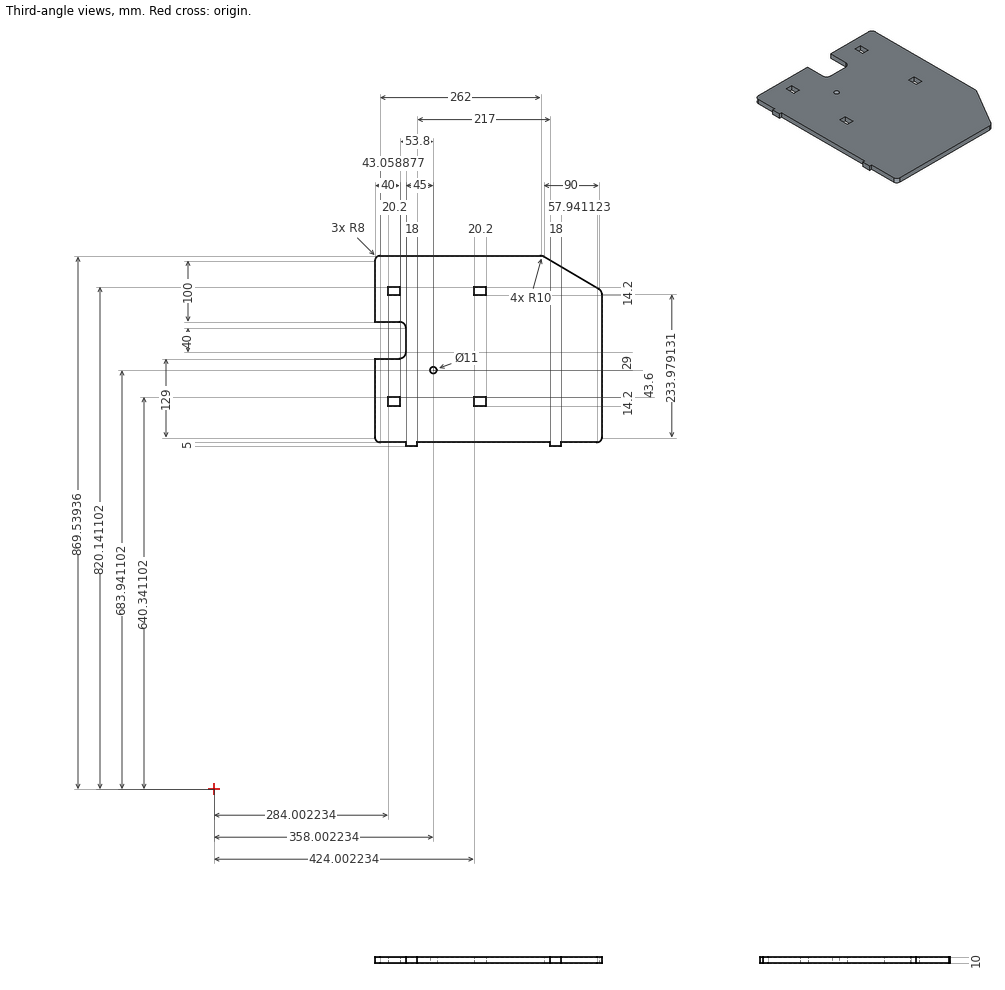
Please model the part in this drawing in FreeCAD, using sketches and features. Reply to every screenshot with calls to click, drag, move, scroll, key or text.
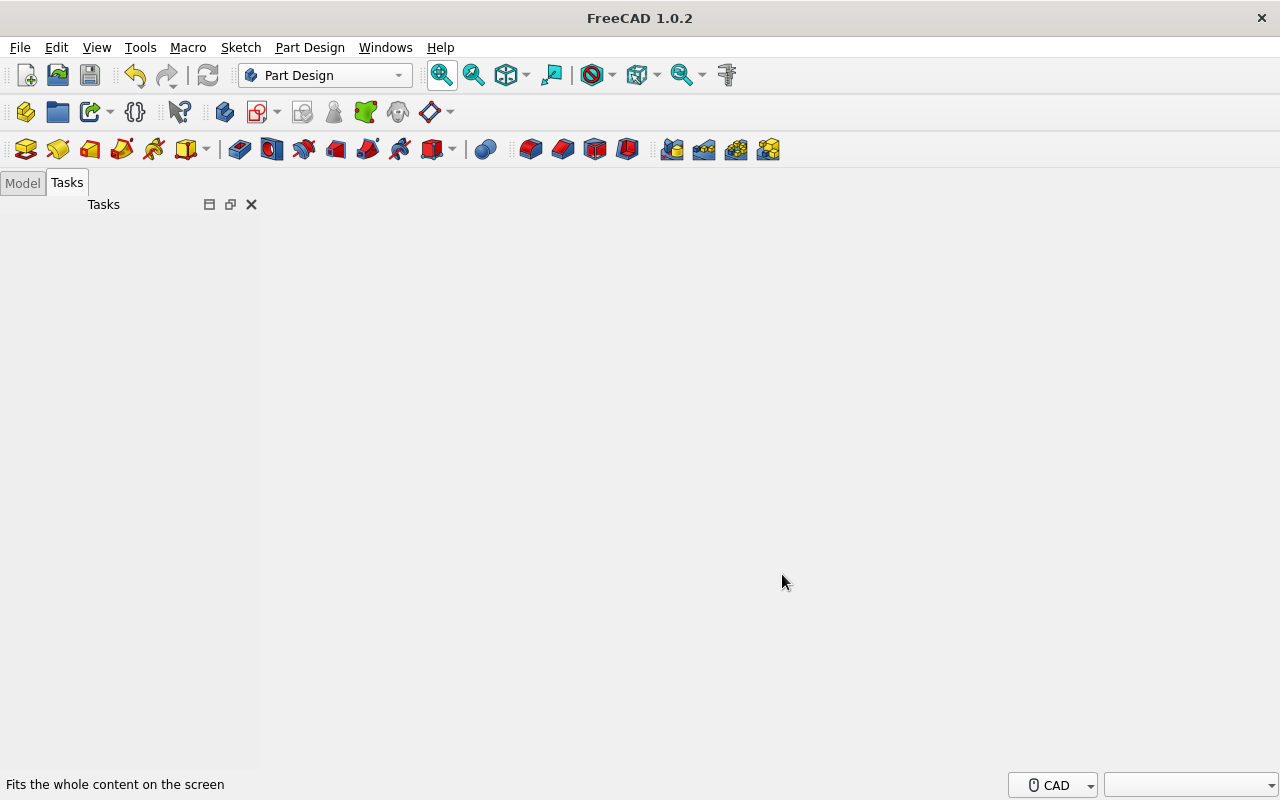
click(26, 76)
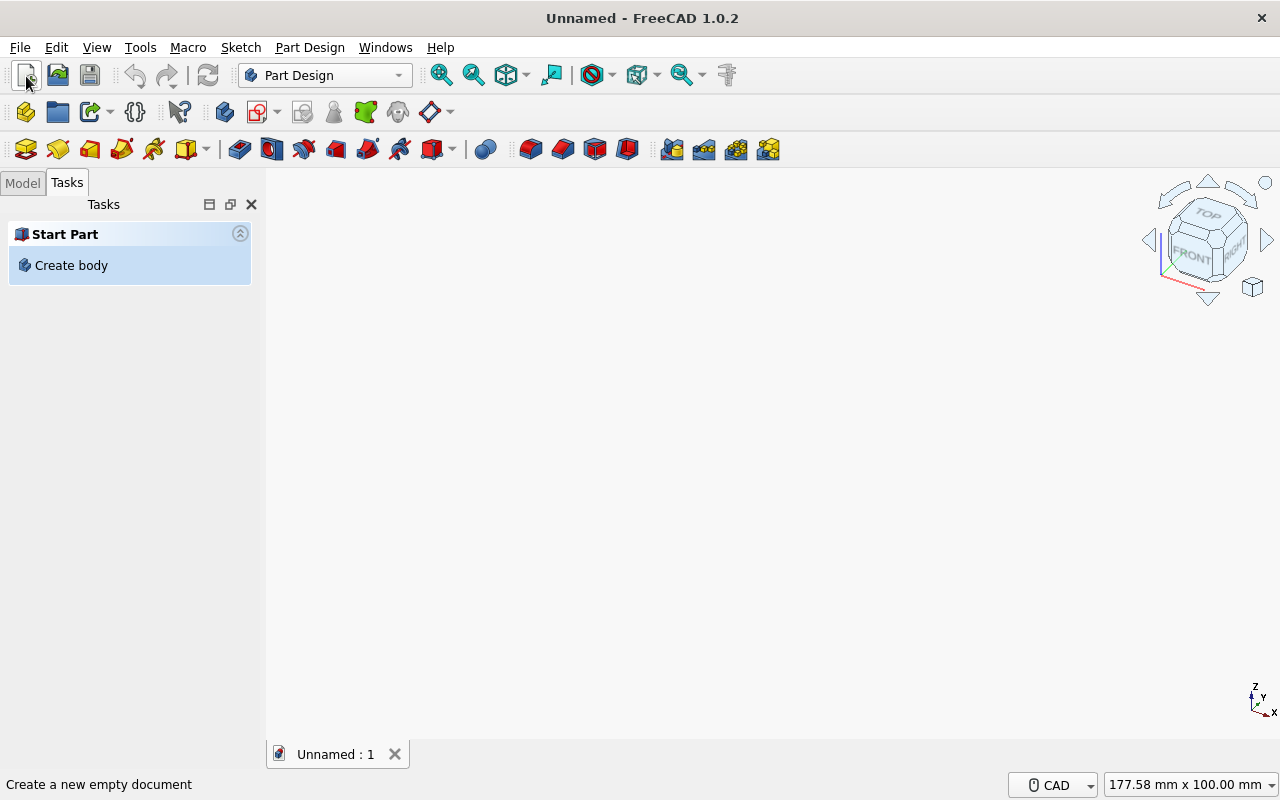
click(258, 112)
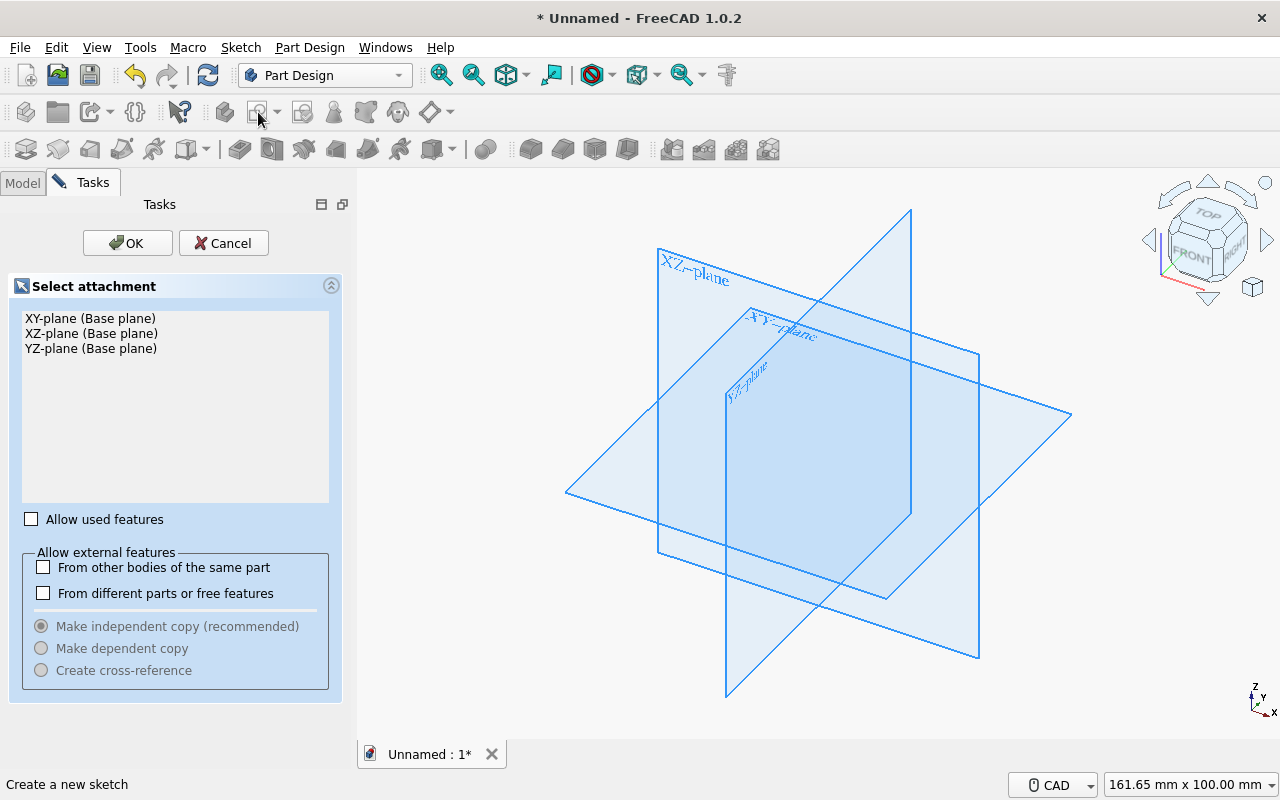
click(82, 318)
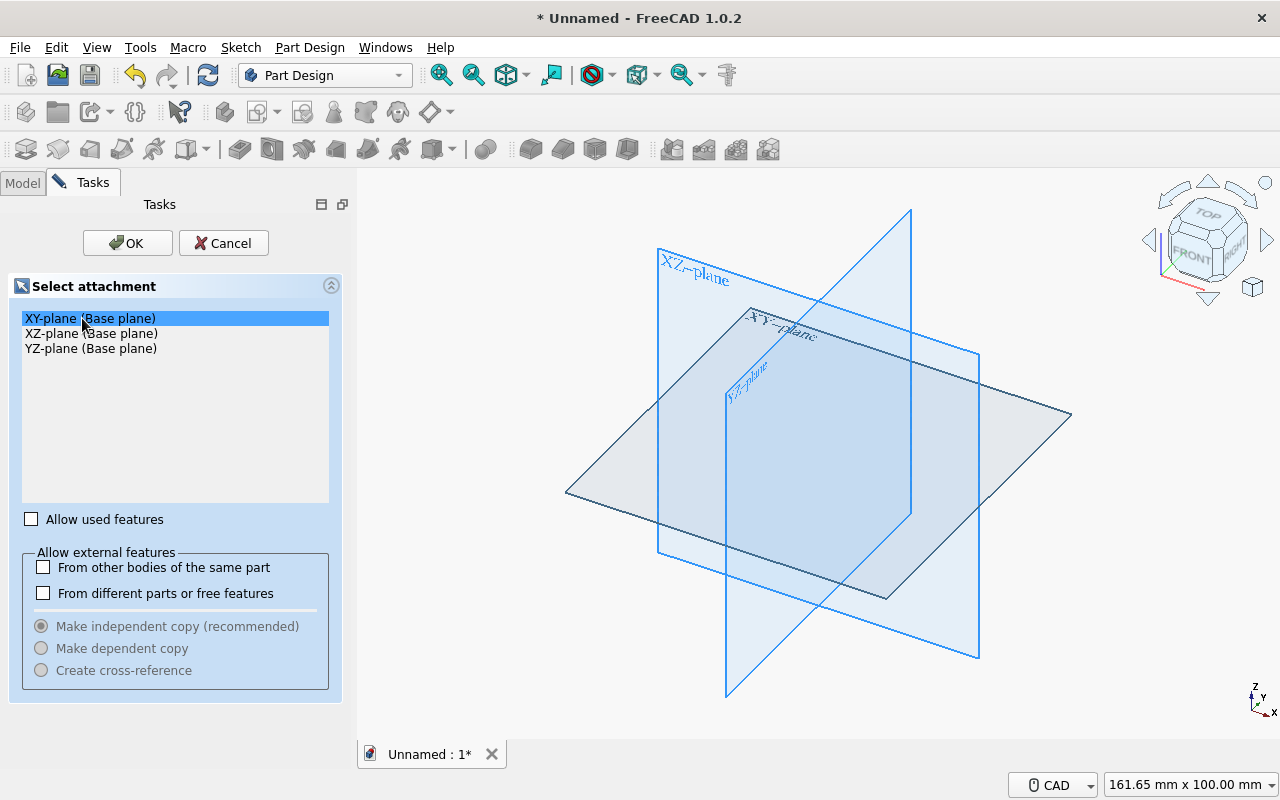
click(128, 243)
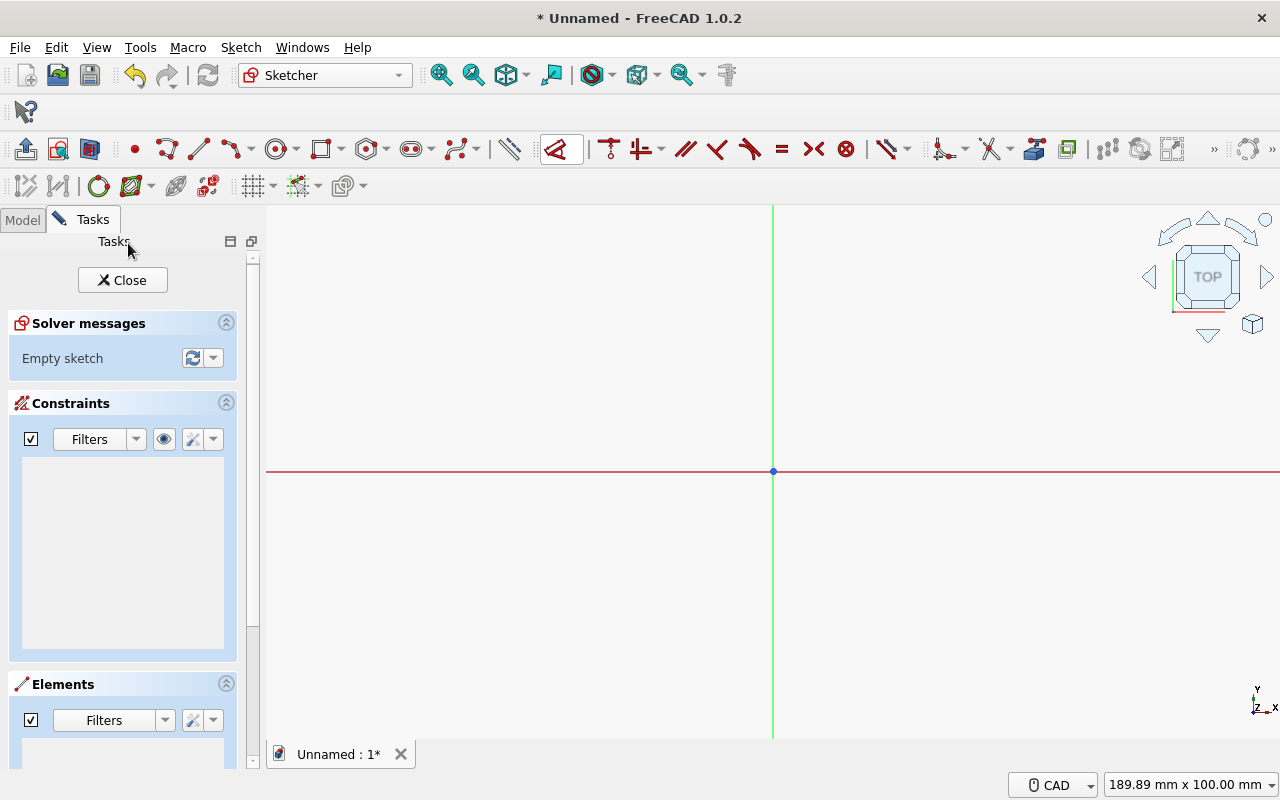
scroll(563, 659, down, 13)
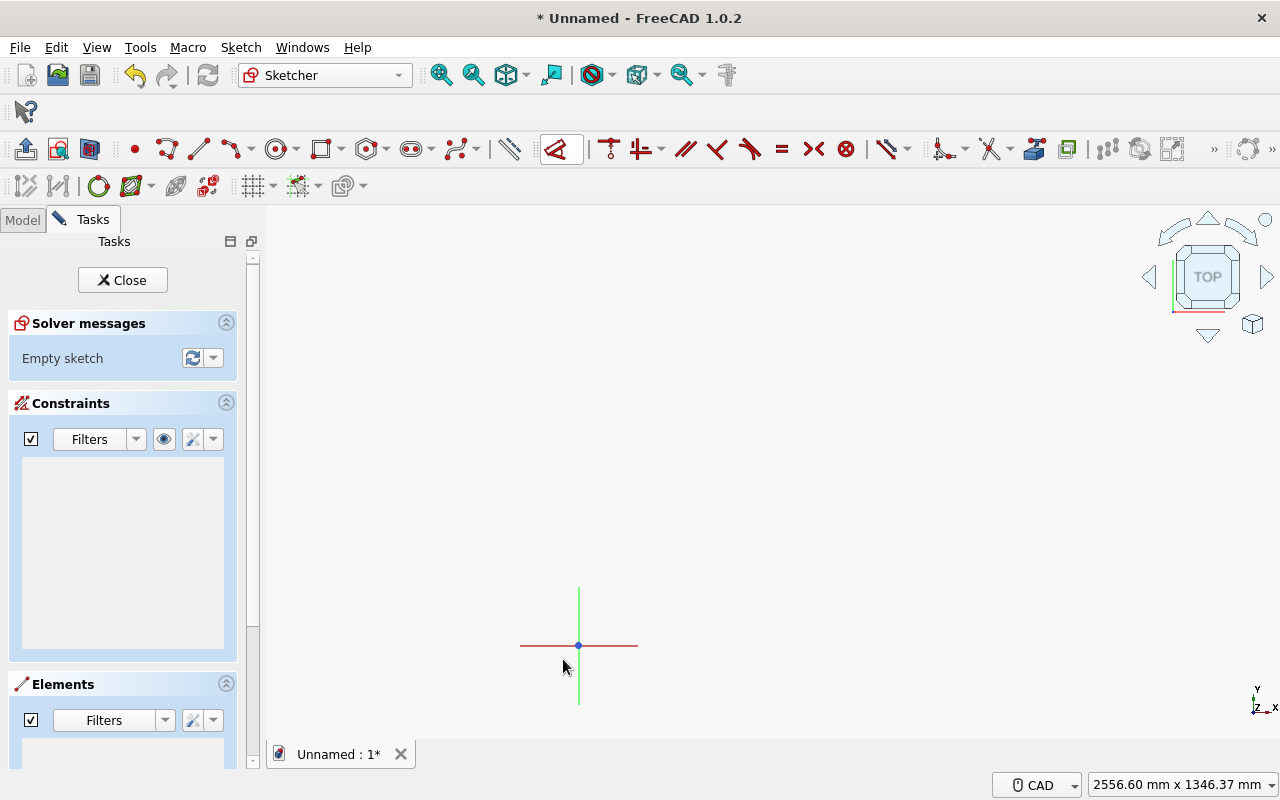
click(200, 150)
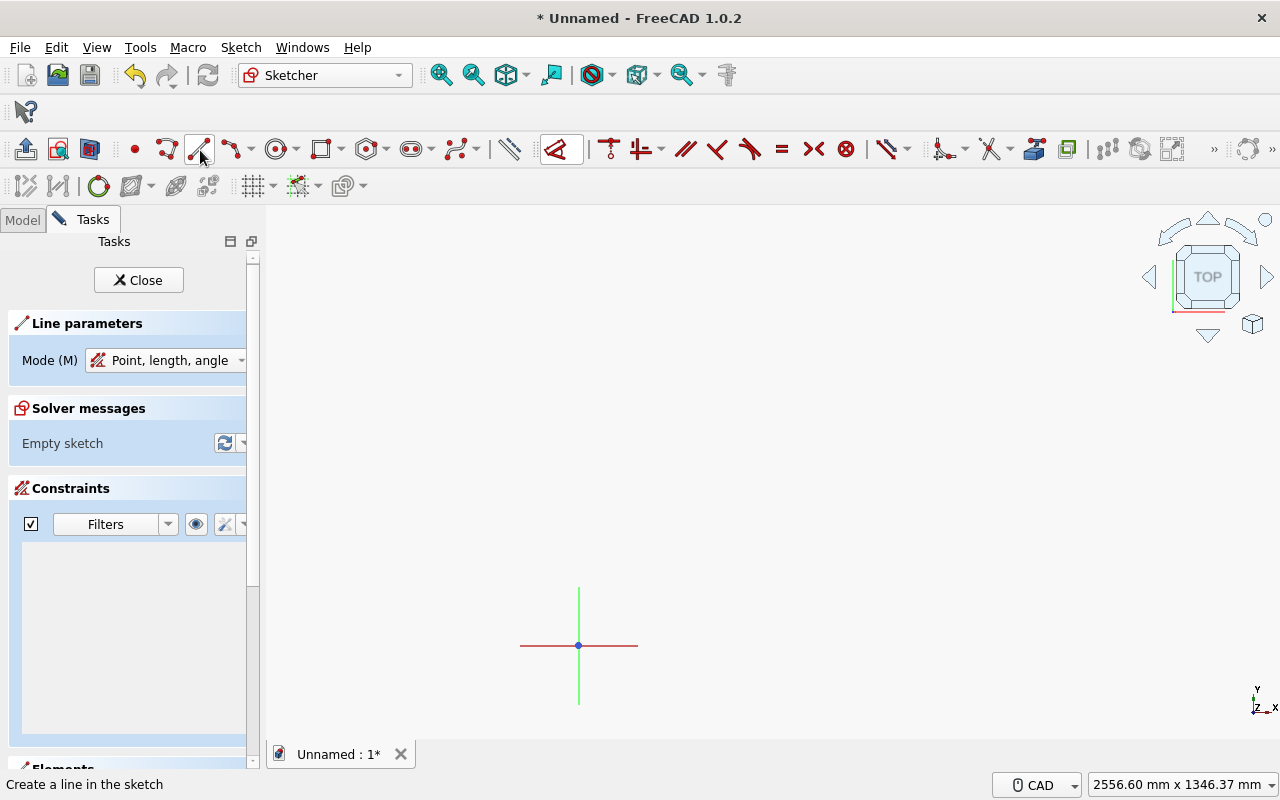
click(828, 322)
click(792, 301)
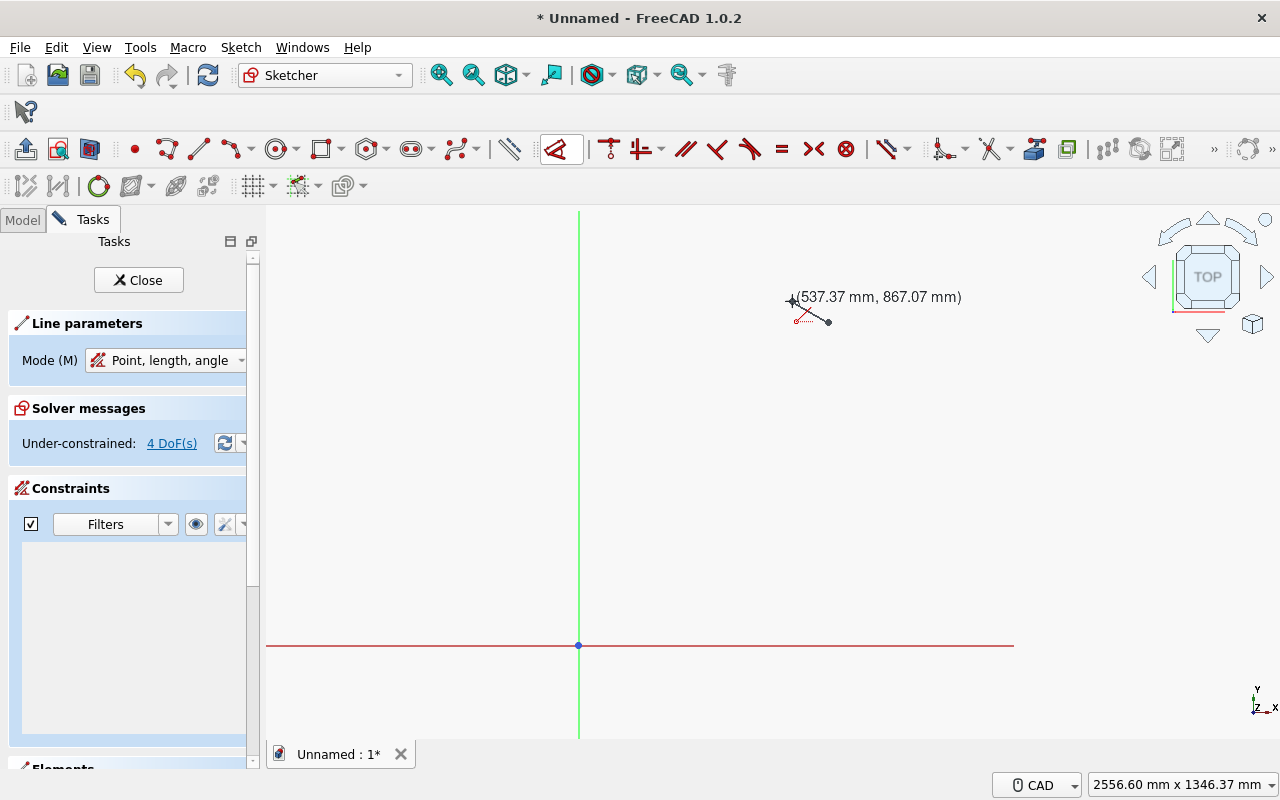
scroll(790, 300, up, 11)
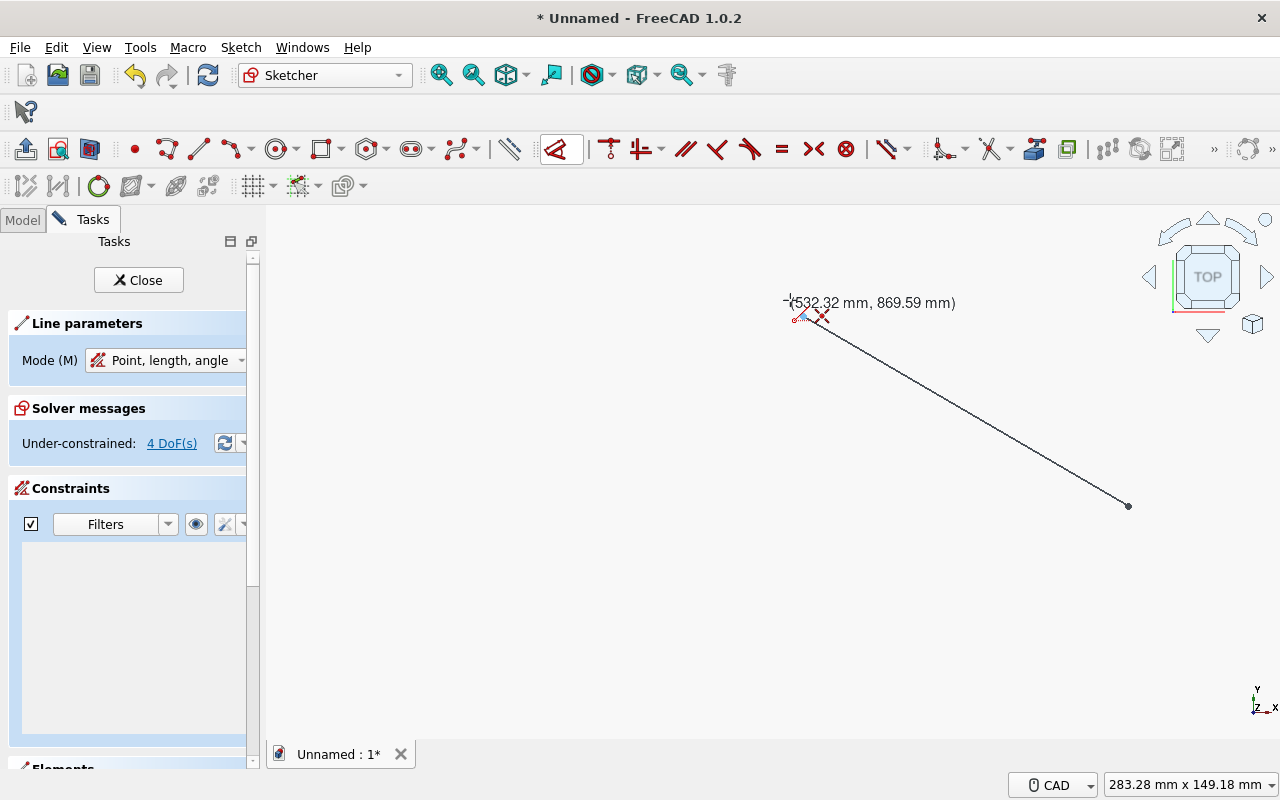
click(788, 303)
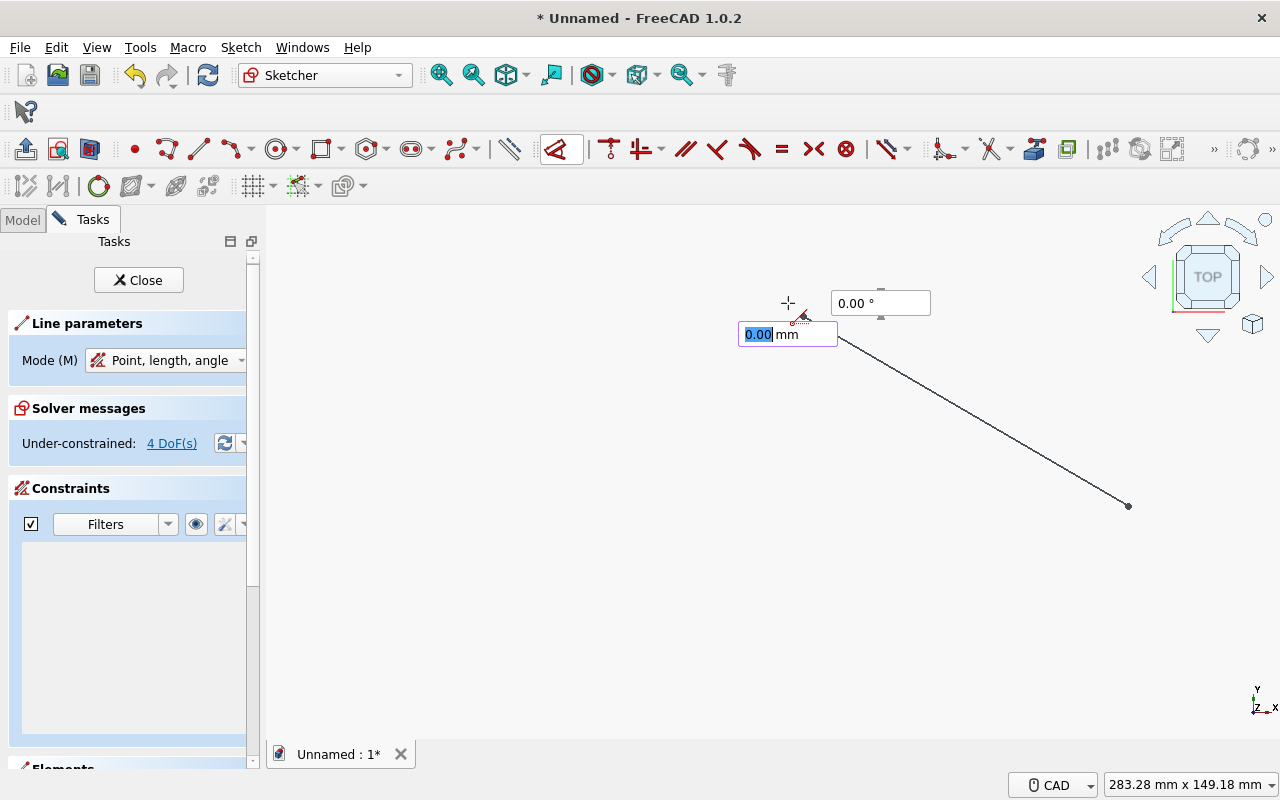
scroll(791, 299, down, 11)